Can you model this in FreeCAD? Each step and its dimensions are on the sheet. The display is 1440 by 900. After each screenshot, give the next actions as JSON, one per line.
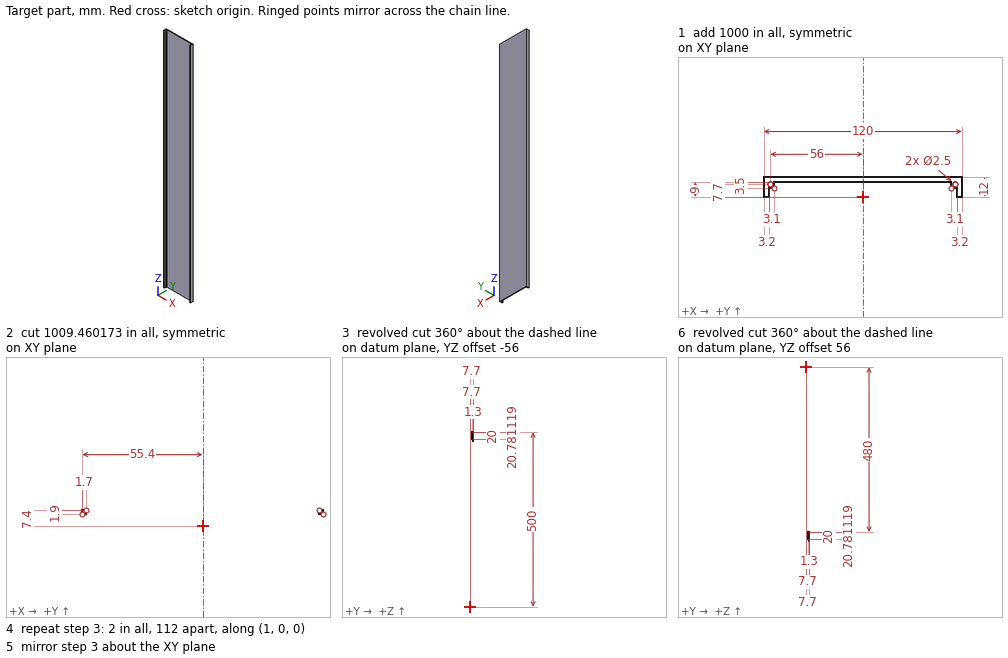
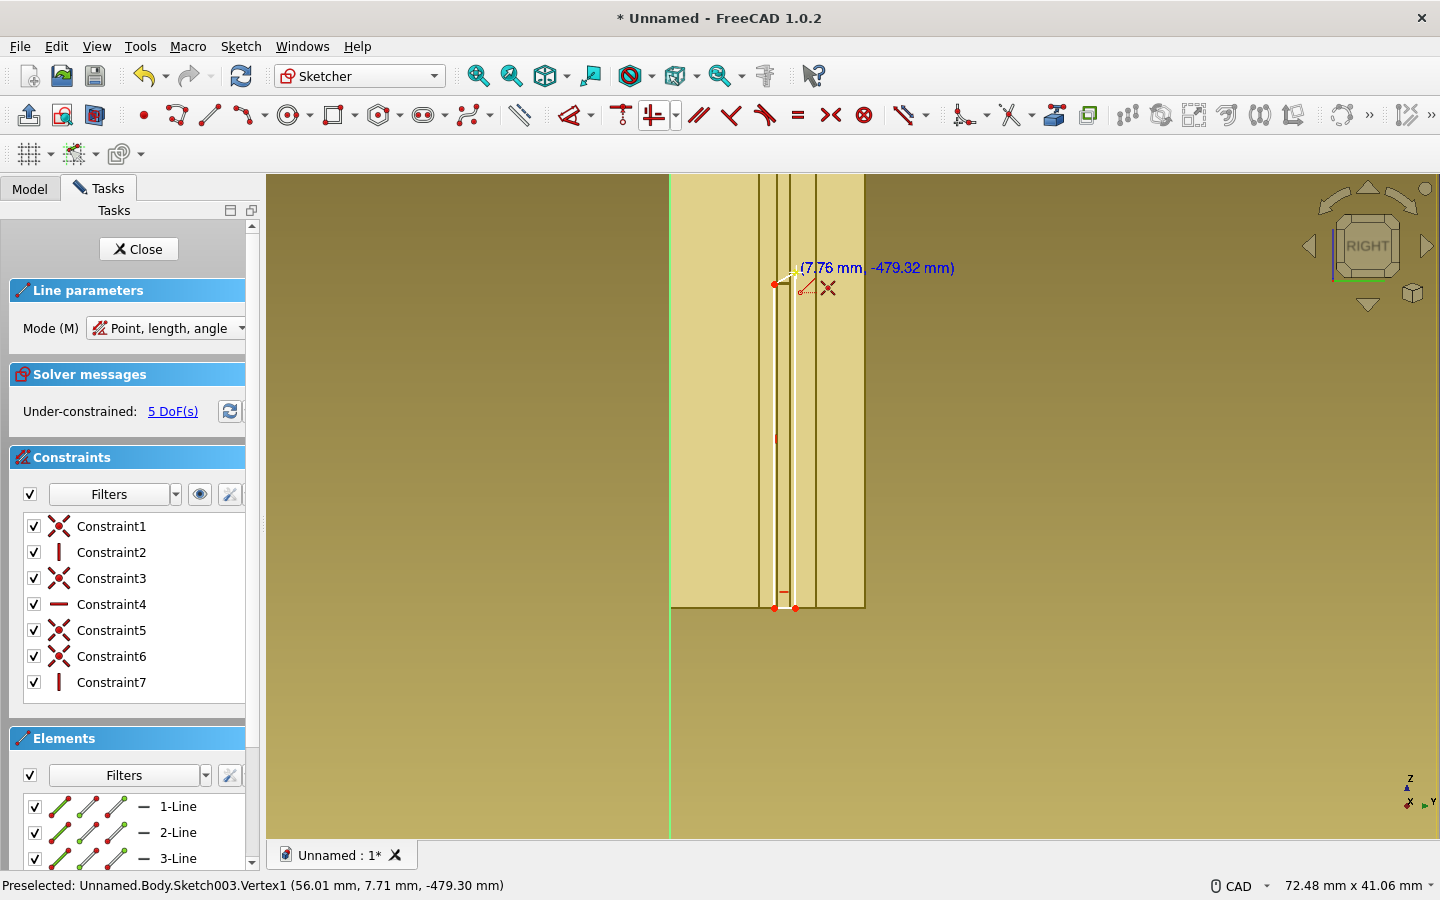
{"action": "left_click", "coordinate": [795, 641]}
{"action": "left_click", "coordinate": [795, 742]}
{"action": "key", "text": "Escape"}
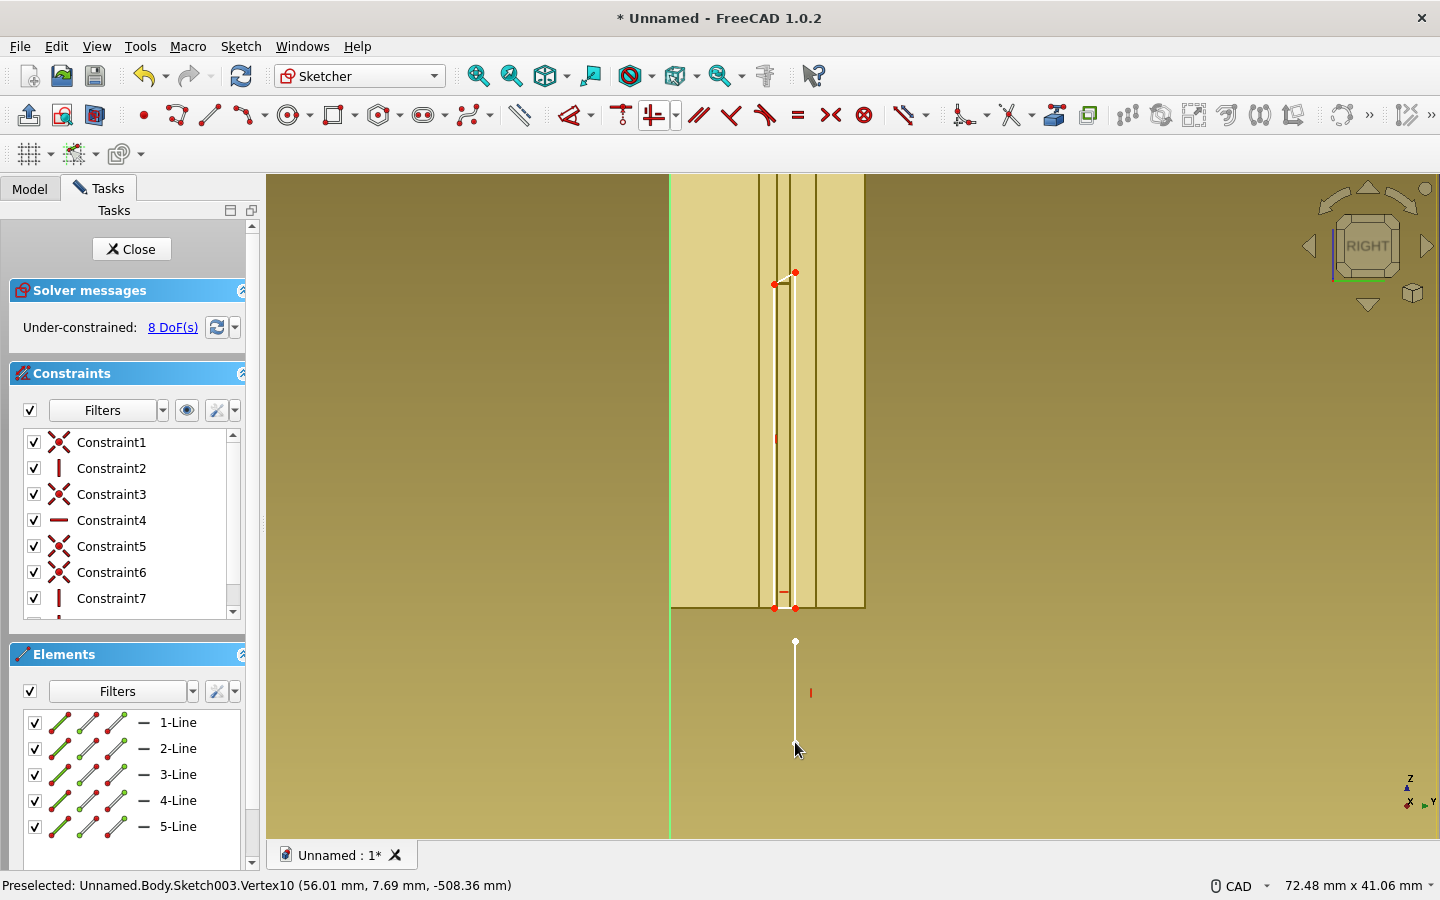
{"action": "left_click", "coordinate": [795, 672]}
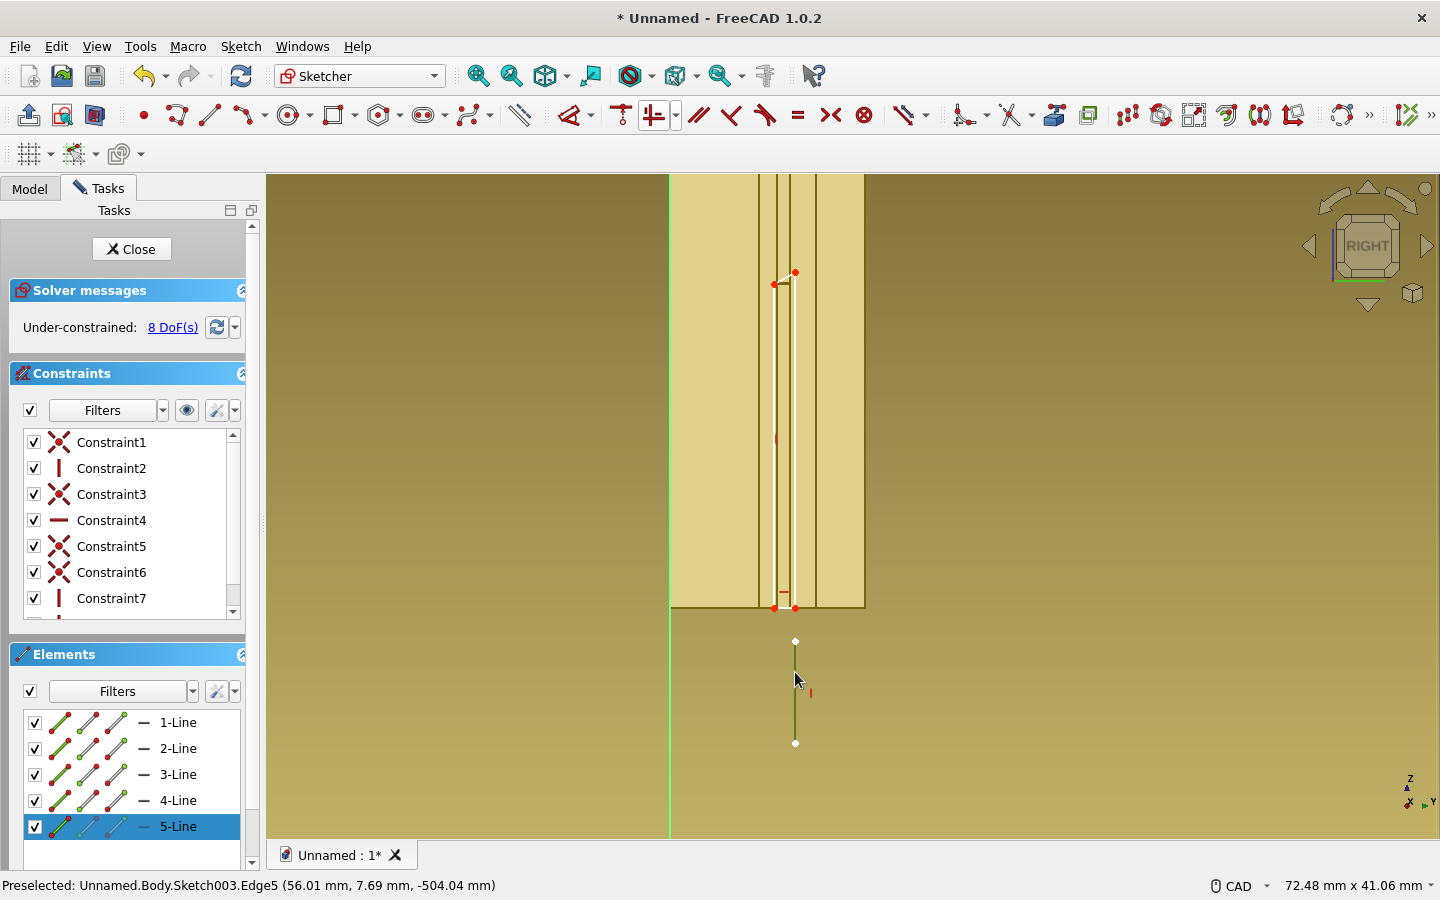
{"action": "key", "text": "g n"}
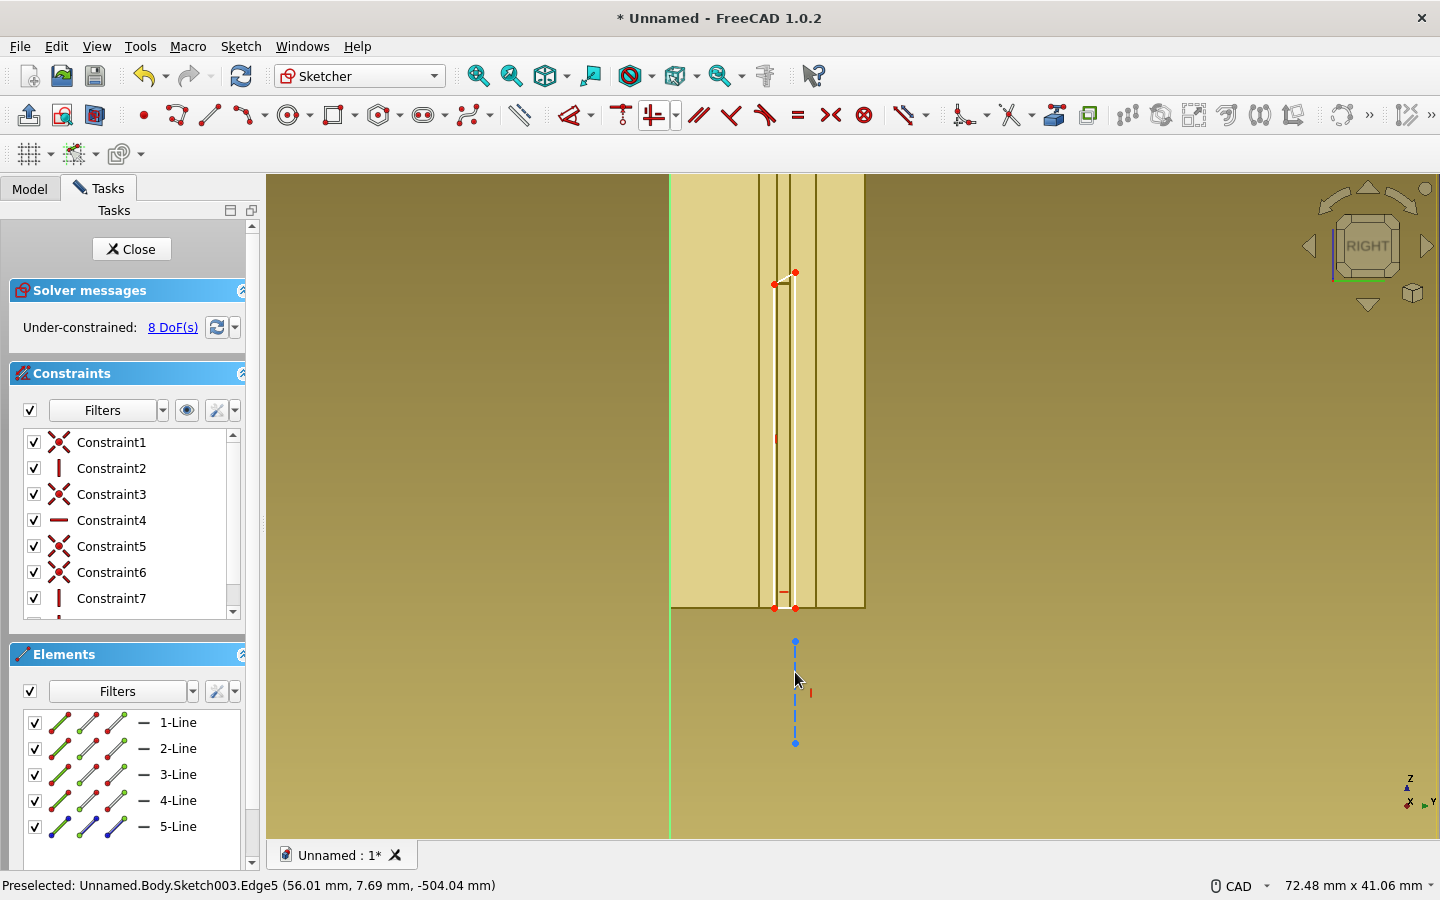
{"action": "left_click", "coordinate": [568, 116]}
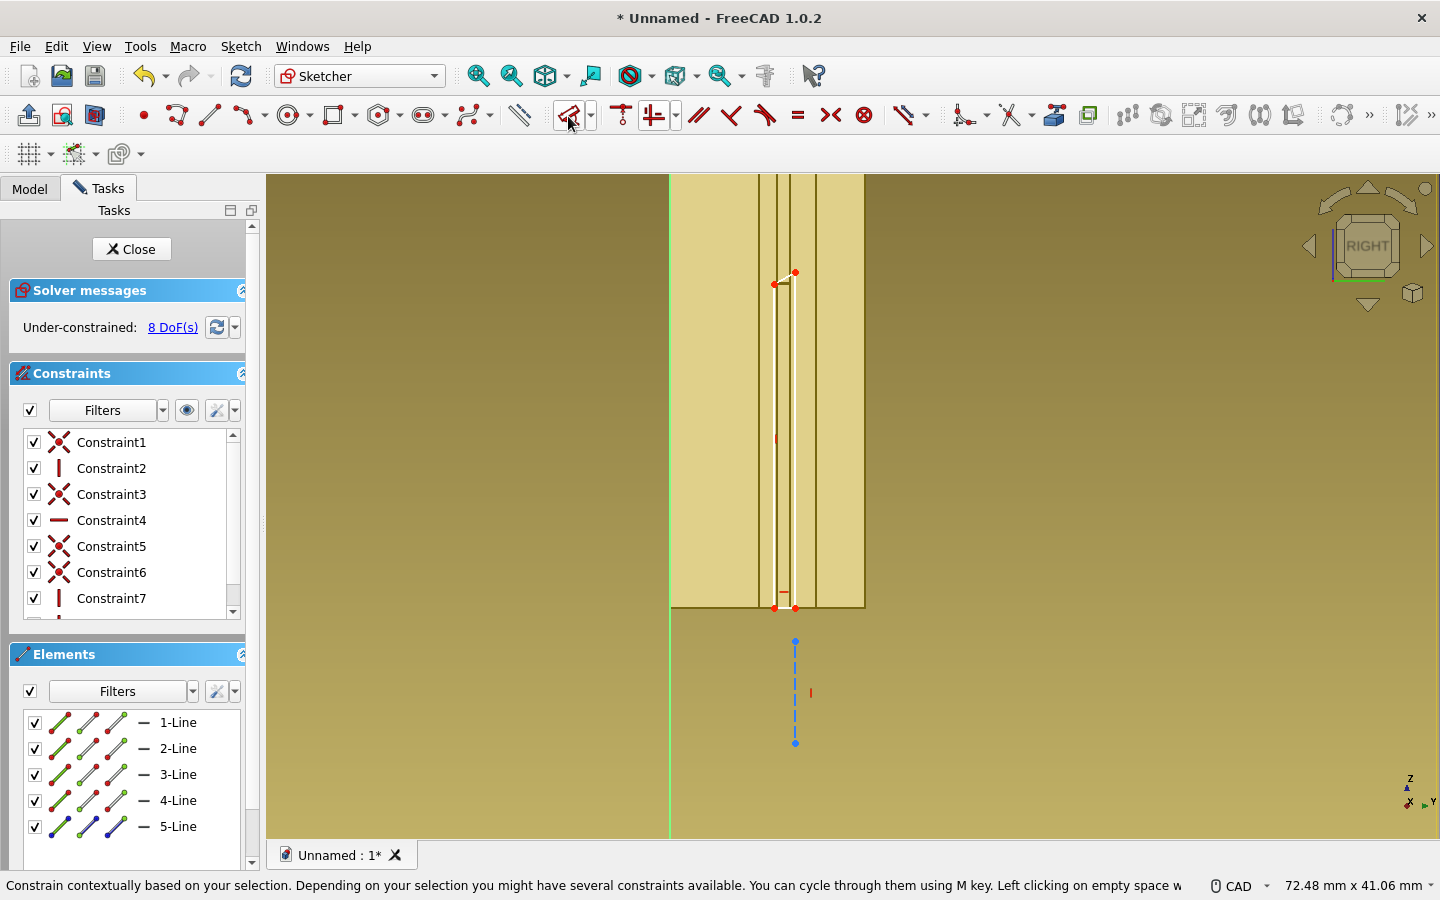
{"action": "left_click", "coordinate": [774, 382]}
{"action": "left_click", "coordinate": [740, 446]}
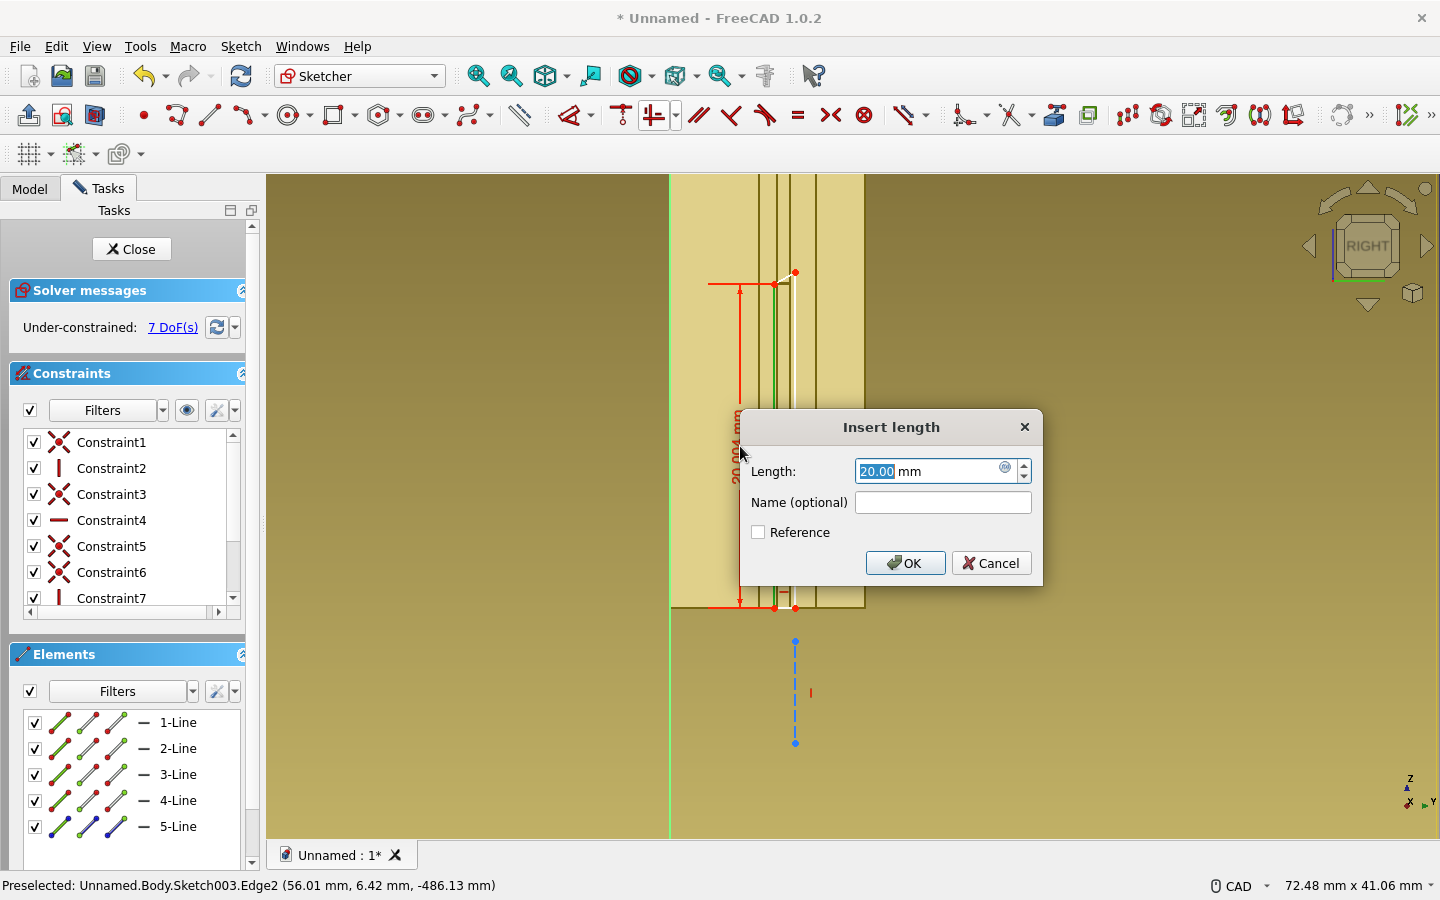
{"action": "type", "text": "20"}
{"action": "key", "text": "Return"}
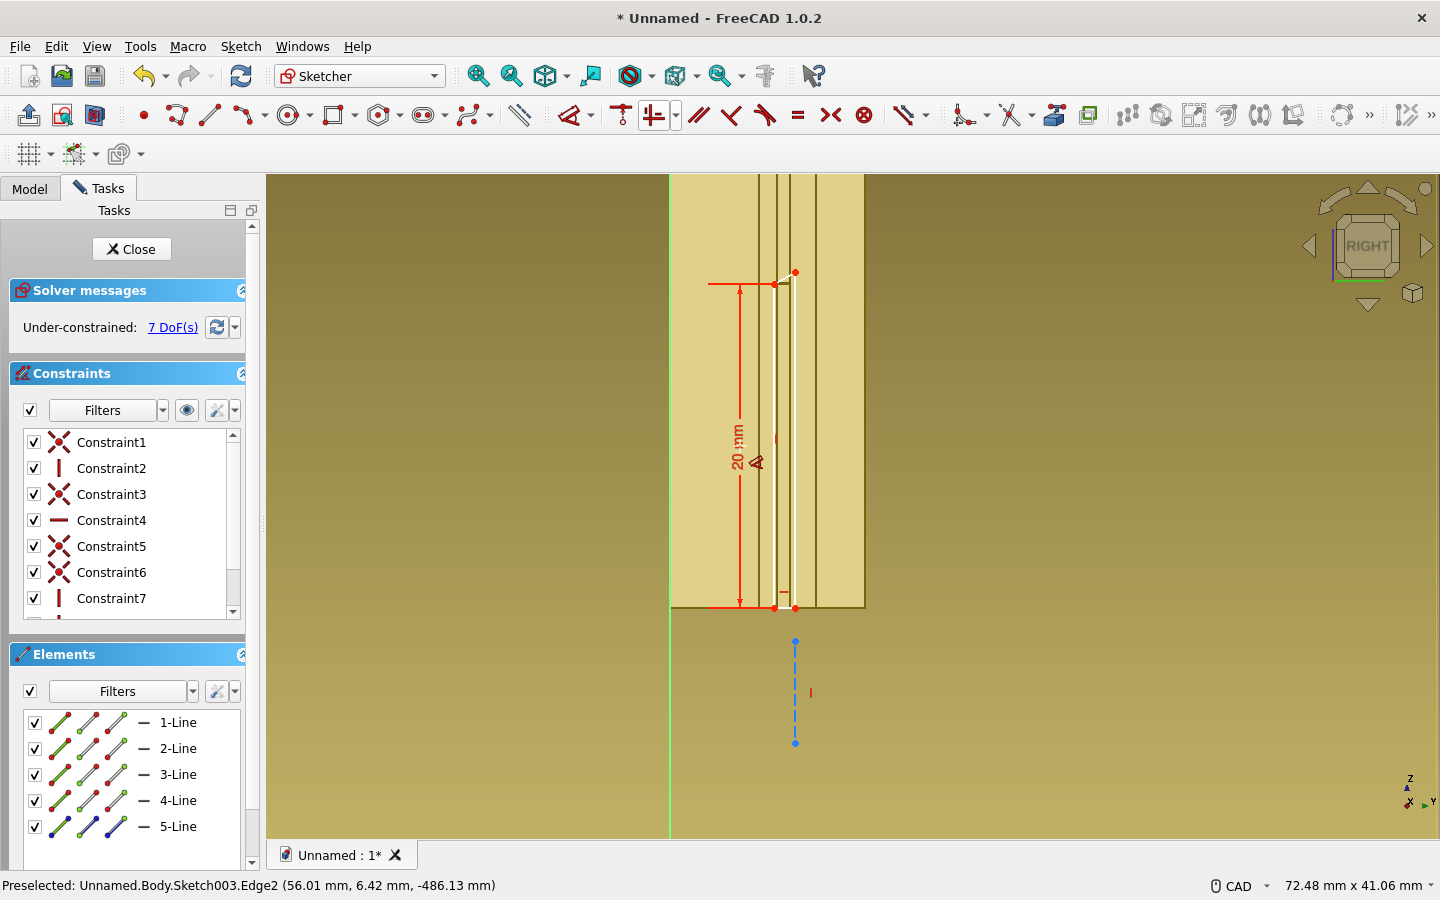
{"action": "scroll", "coordinate": [785, 608], "scroll_direction": "up", "scroll_amount": 4}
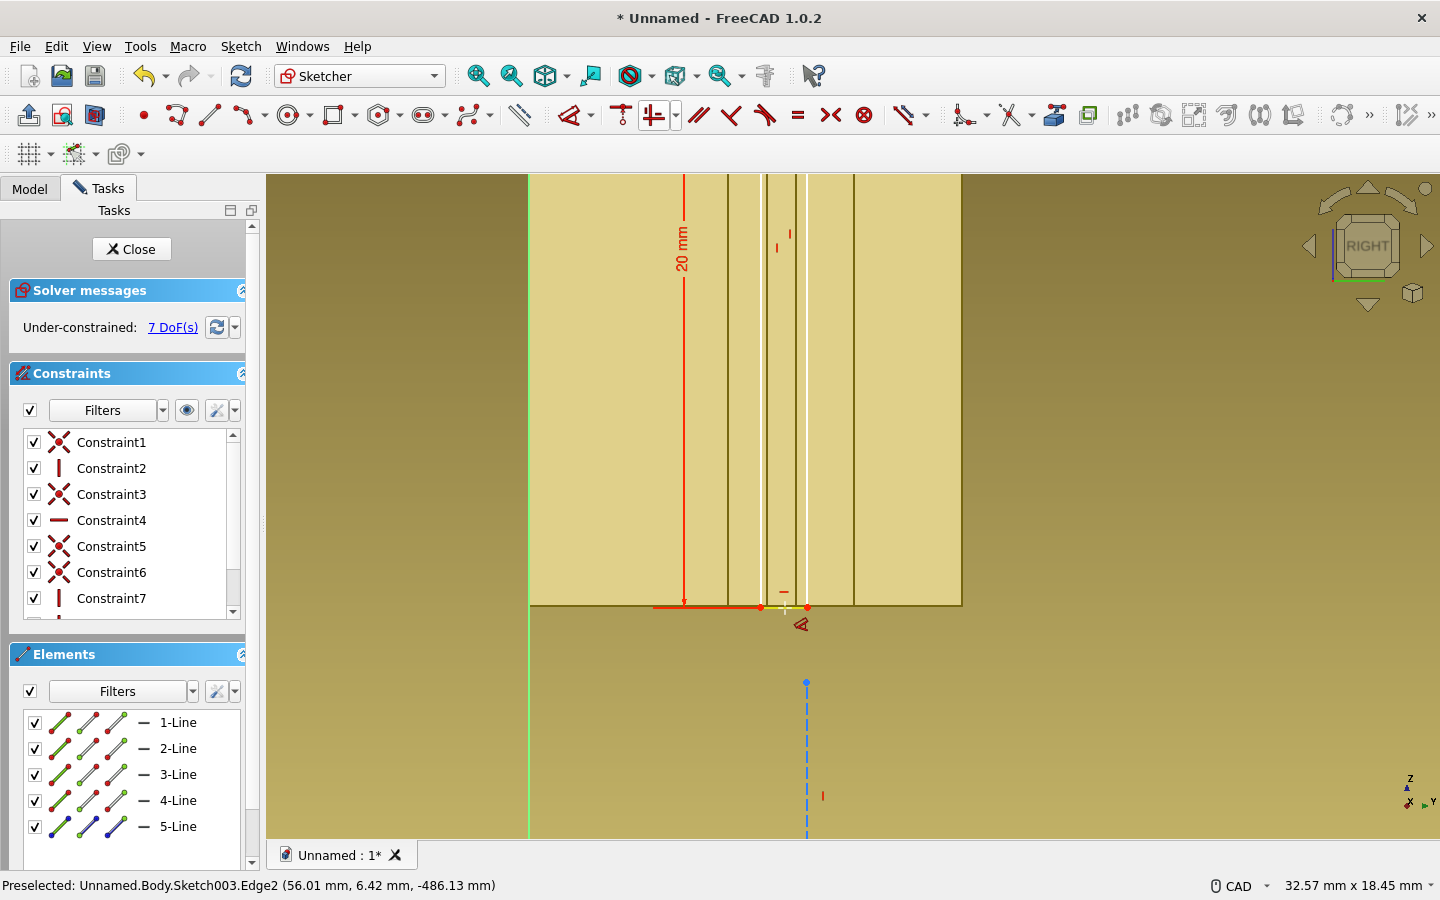
{"action": "left_click", "coordinate": [784, 608]}
{"action": "left_click", "coordinate": [784, 642]}